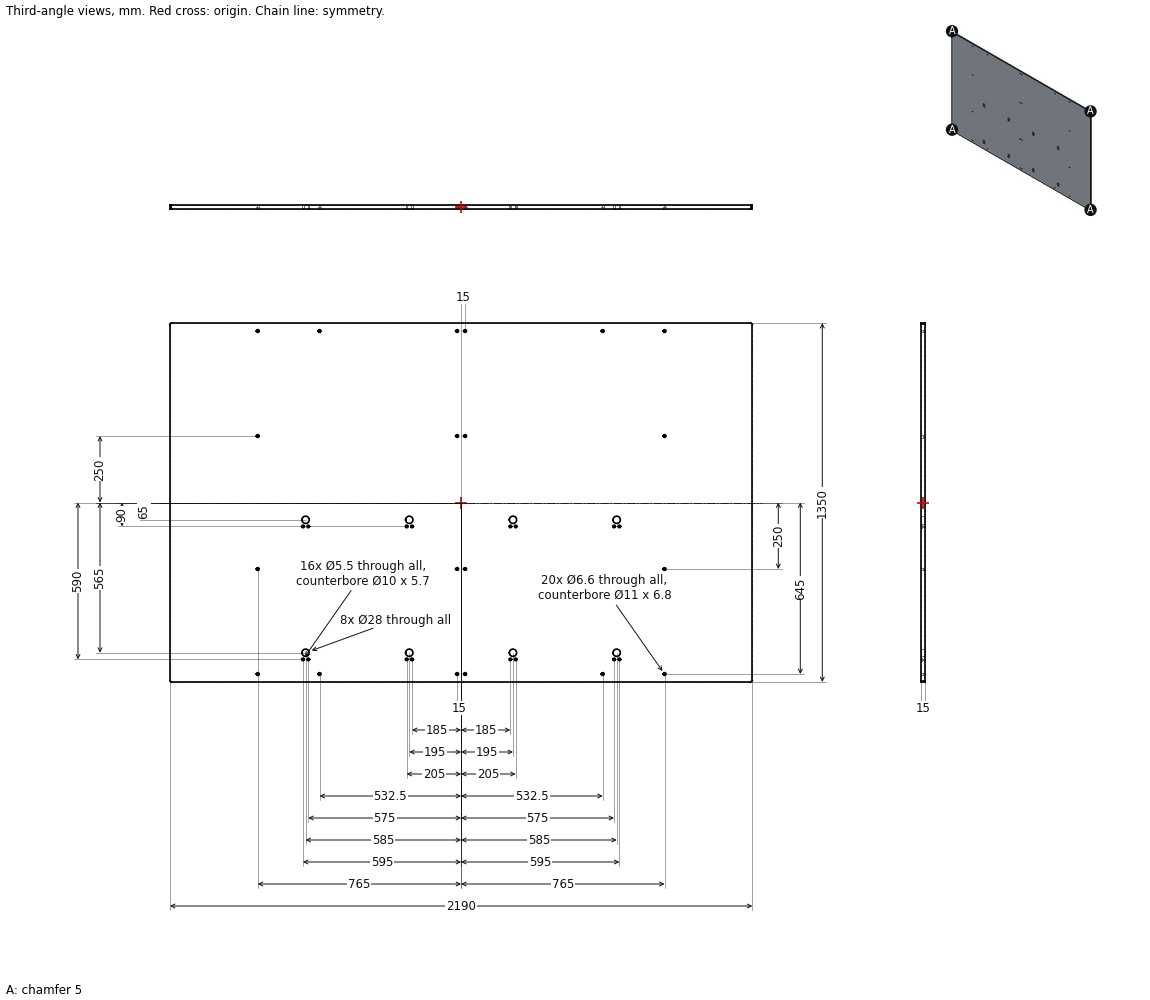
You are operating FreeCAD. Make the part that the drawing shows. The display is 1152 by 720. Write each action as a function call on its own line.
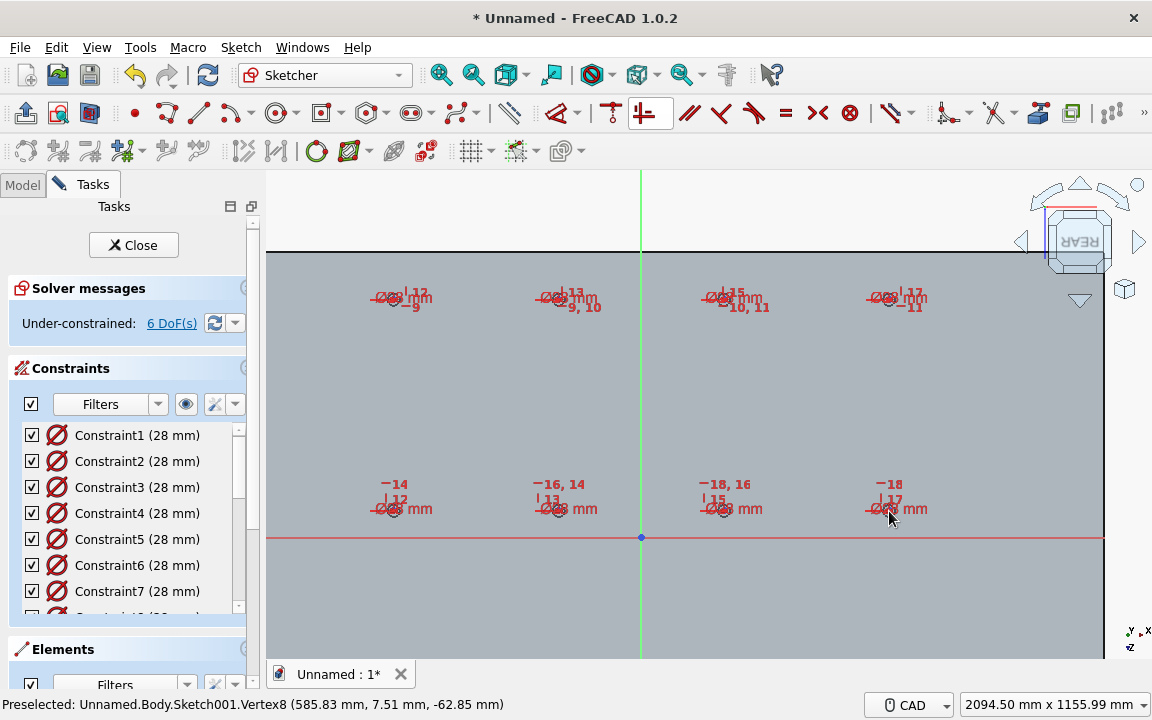
click(556, 114)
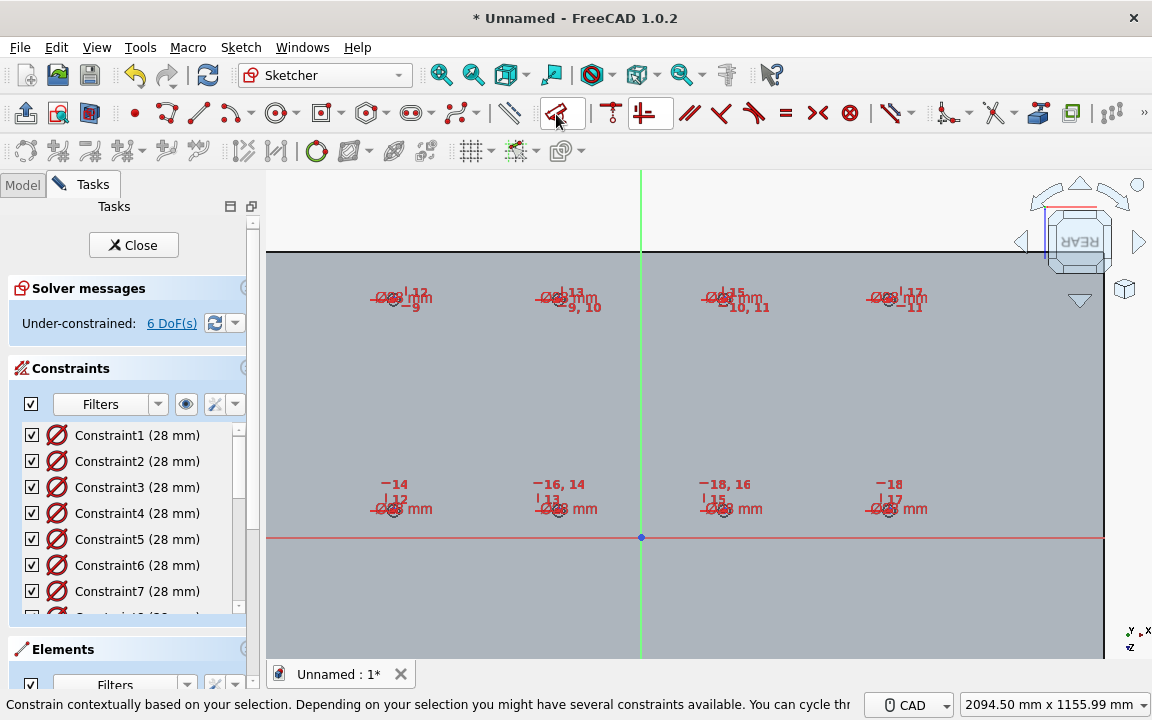
scroll(394, 511, up, 2)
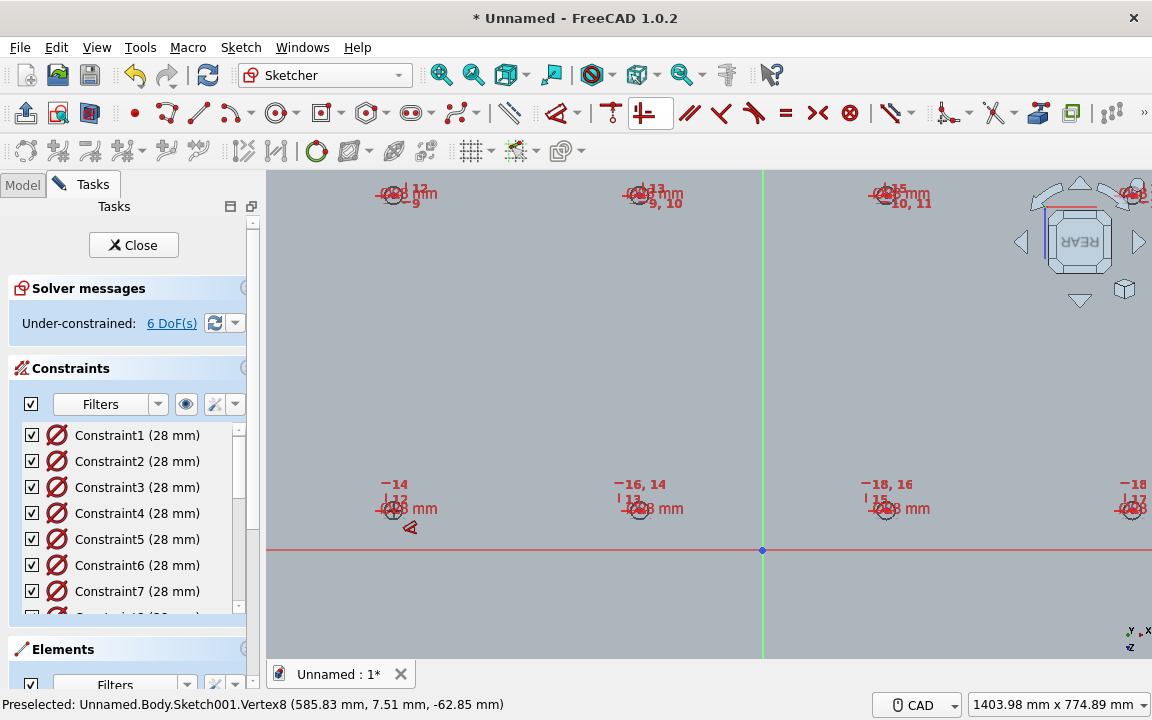
click(394, 511)
click(360, 530)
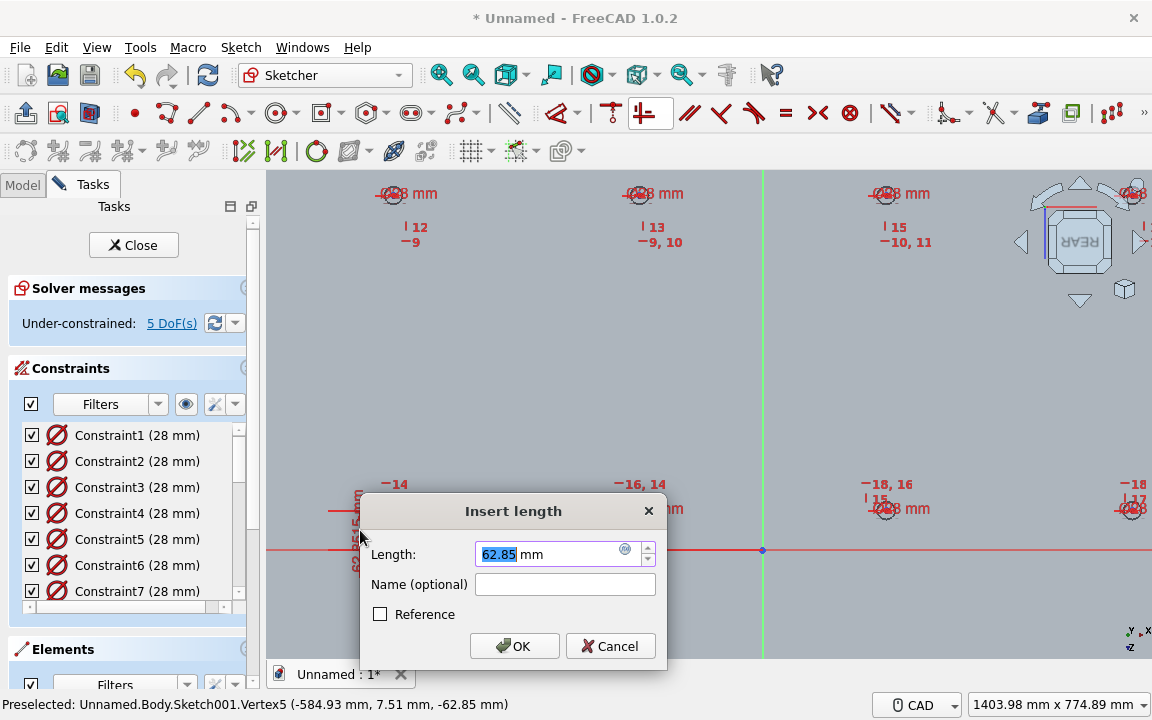
text(65)
key(Return)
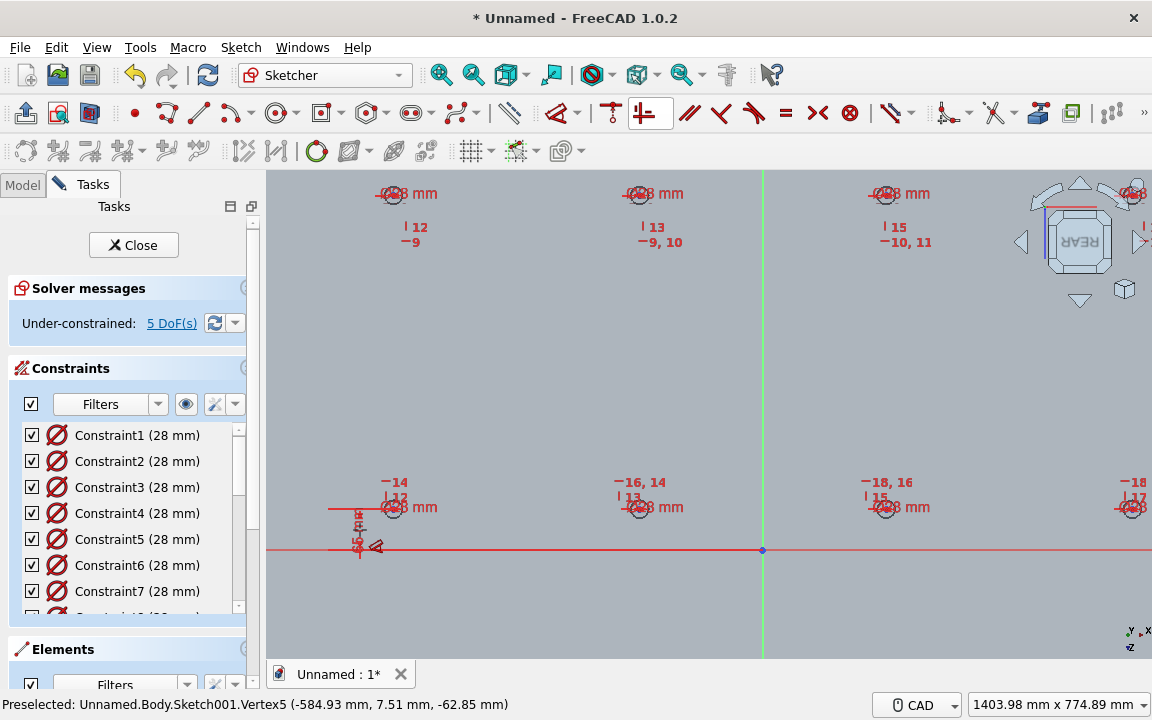
scroll(392, 510, down, 2)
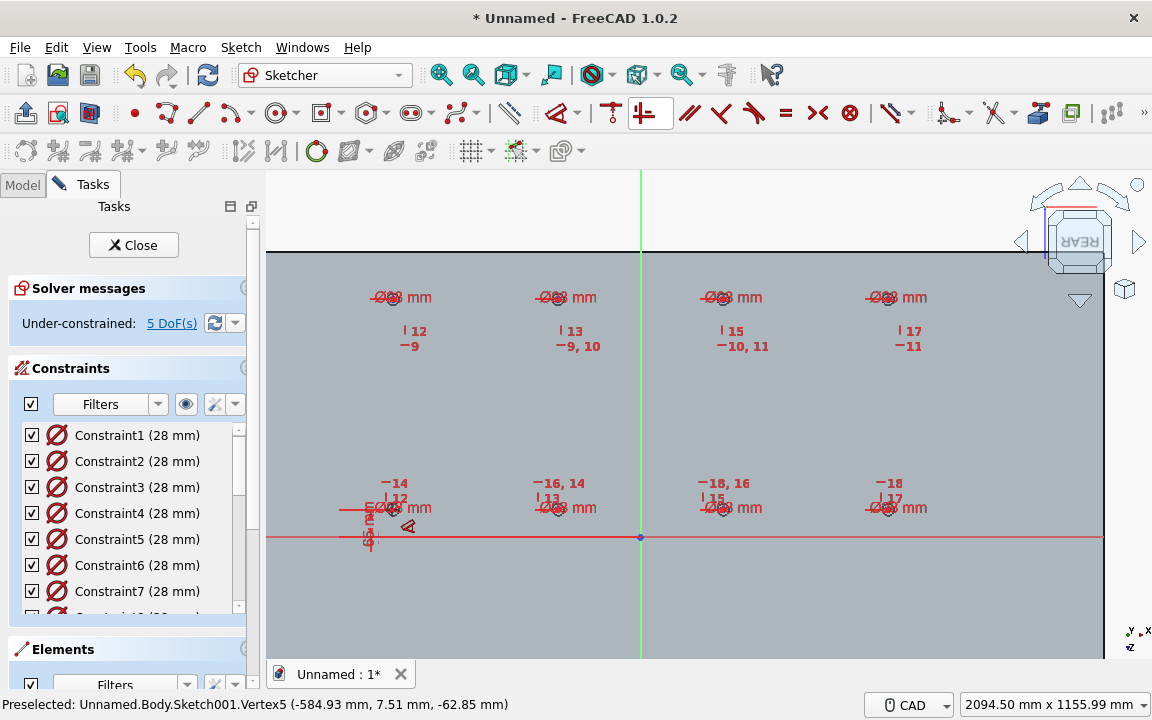
click(393, 299)
click(517, 571)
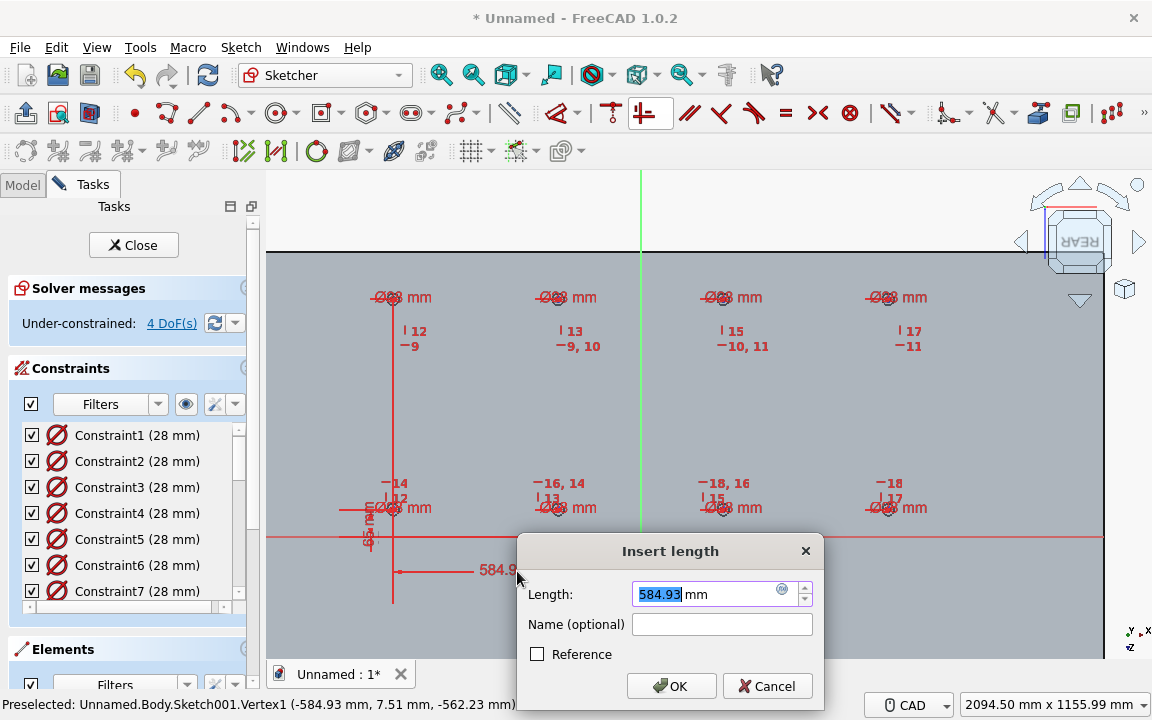
text(585)
key(Return)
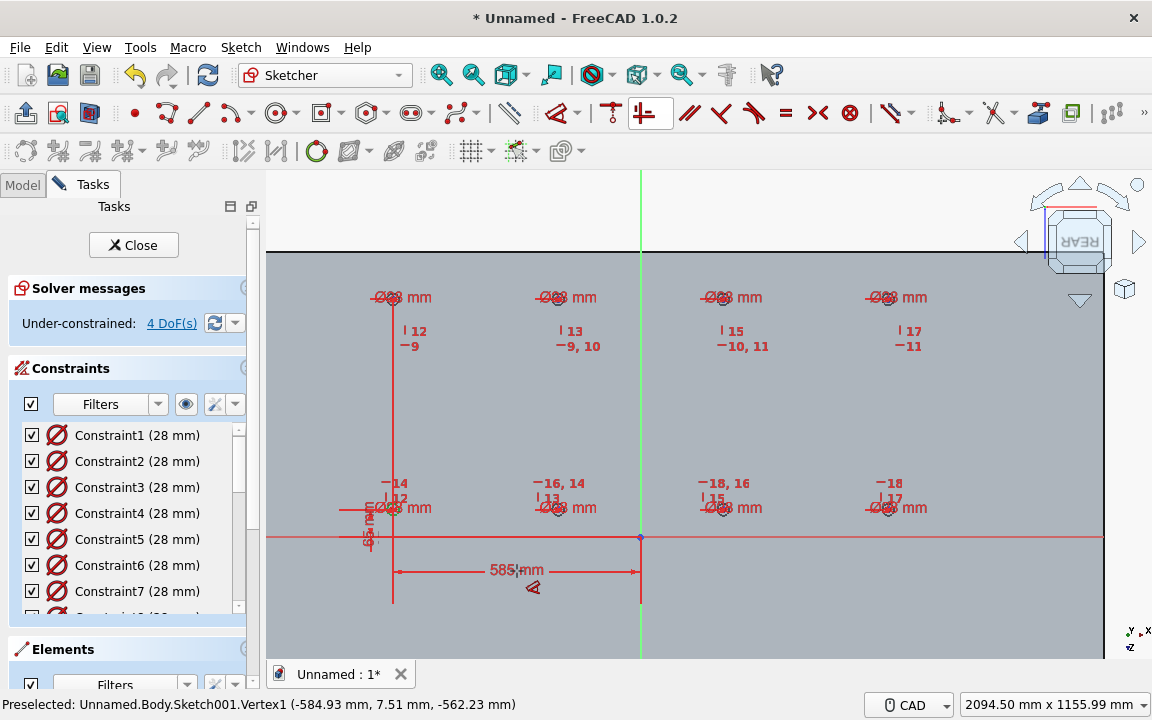
click(393, 299)
click(359, 418)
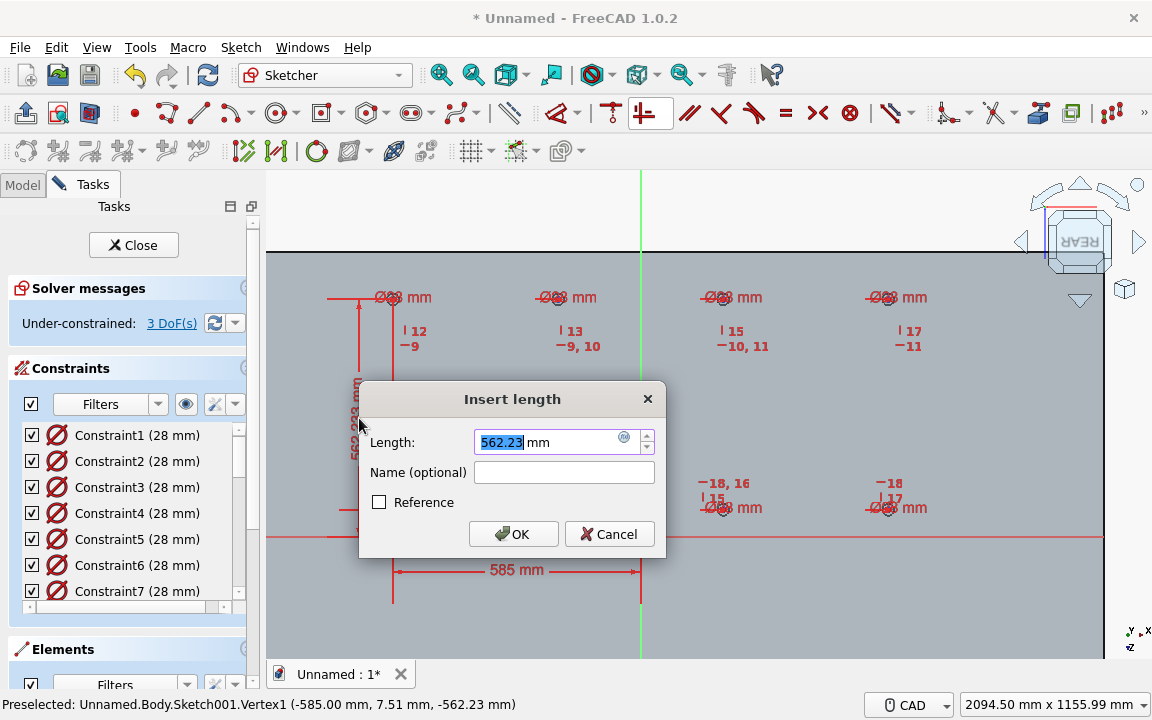
text(565)
key(Return)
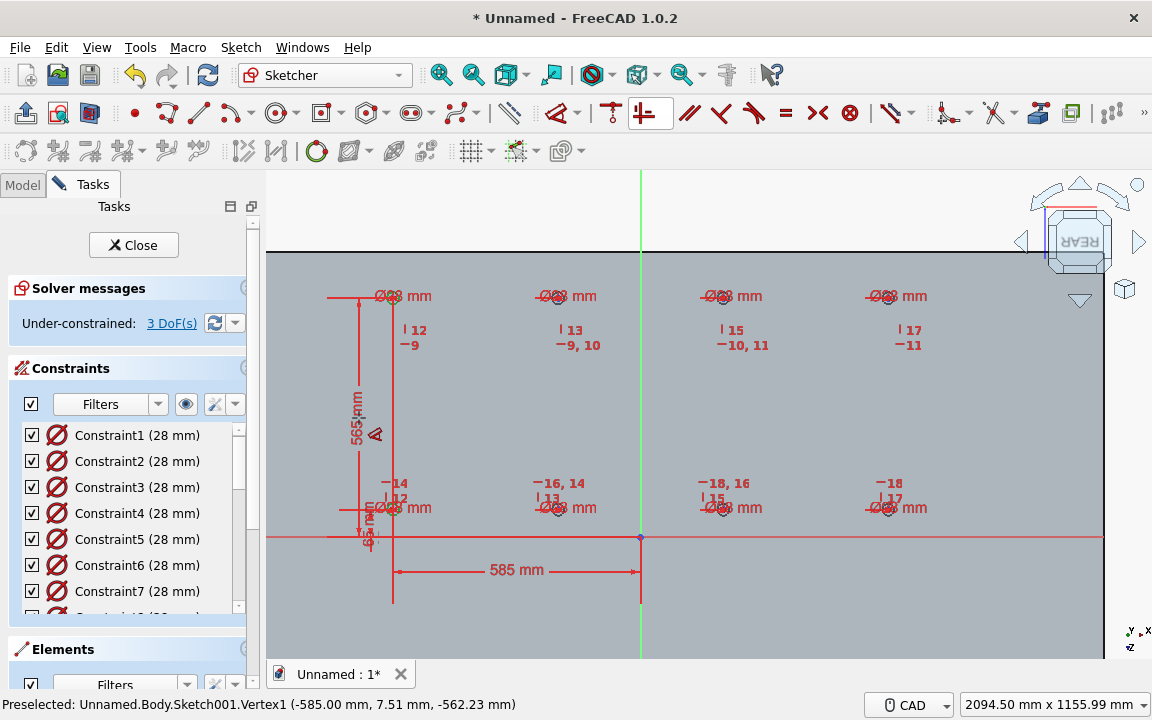
click(558, 298)
click(599, 571)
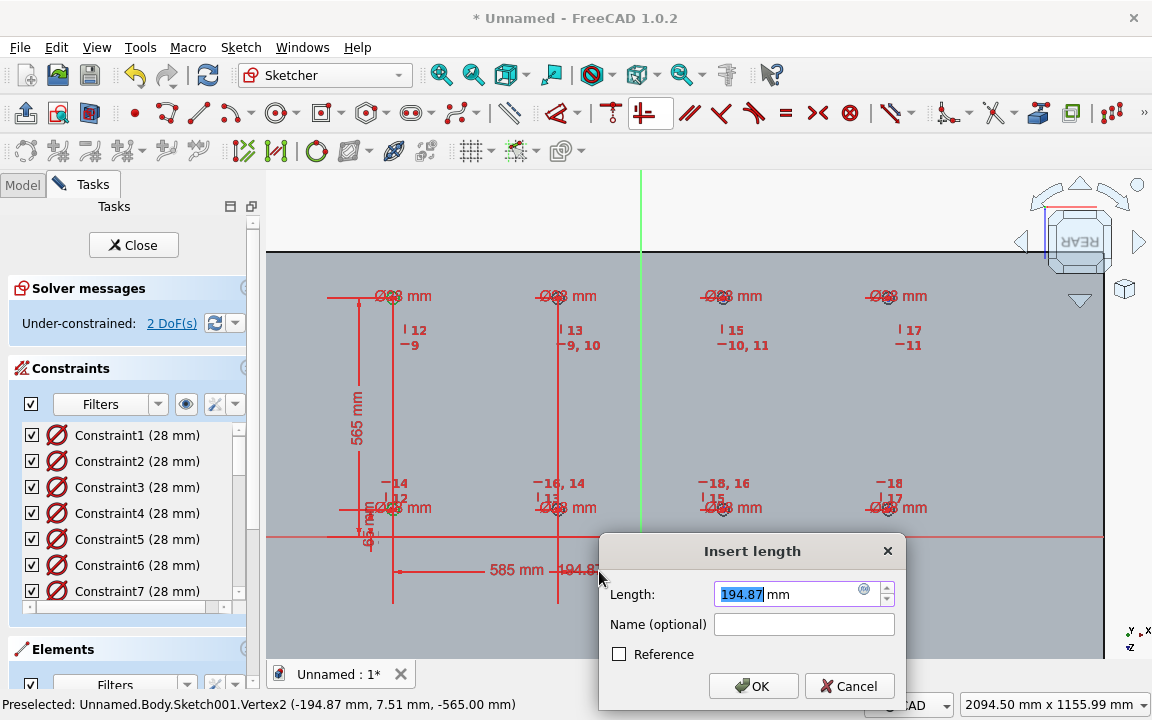
text(195)
key(Return)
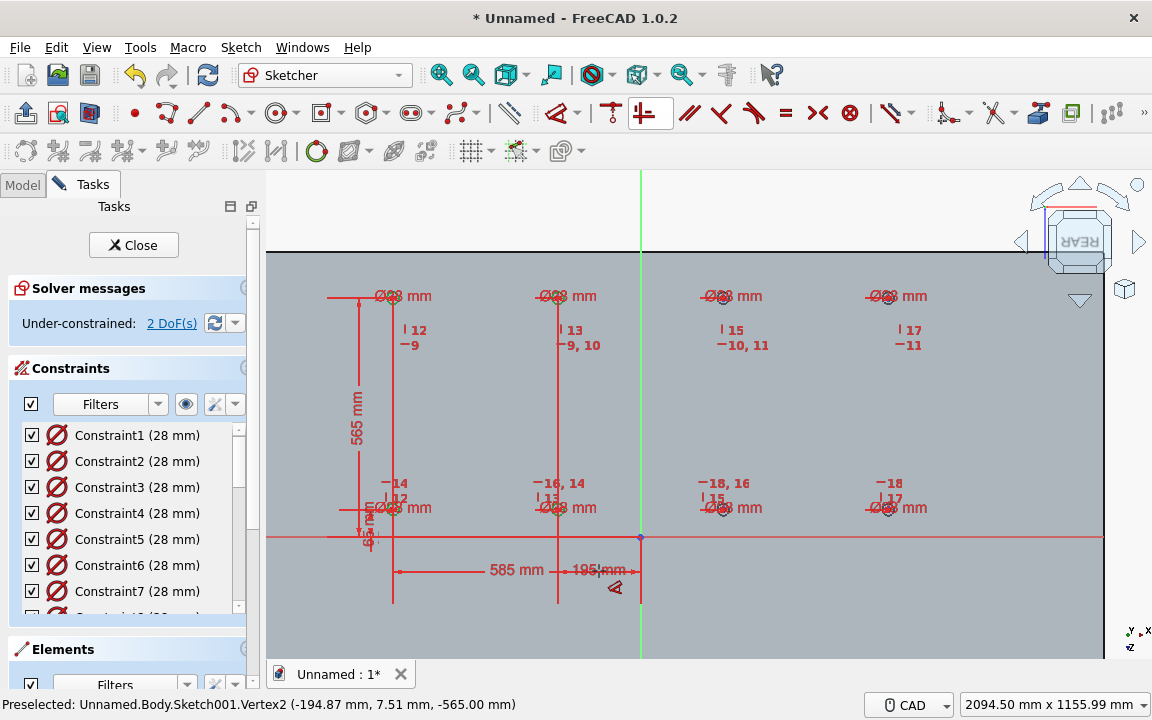
click(723, 298)
click(682, 571)